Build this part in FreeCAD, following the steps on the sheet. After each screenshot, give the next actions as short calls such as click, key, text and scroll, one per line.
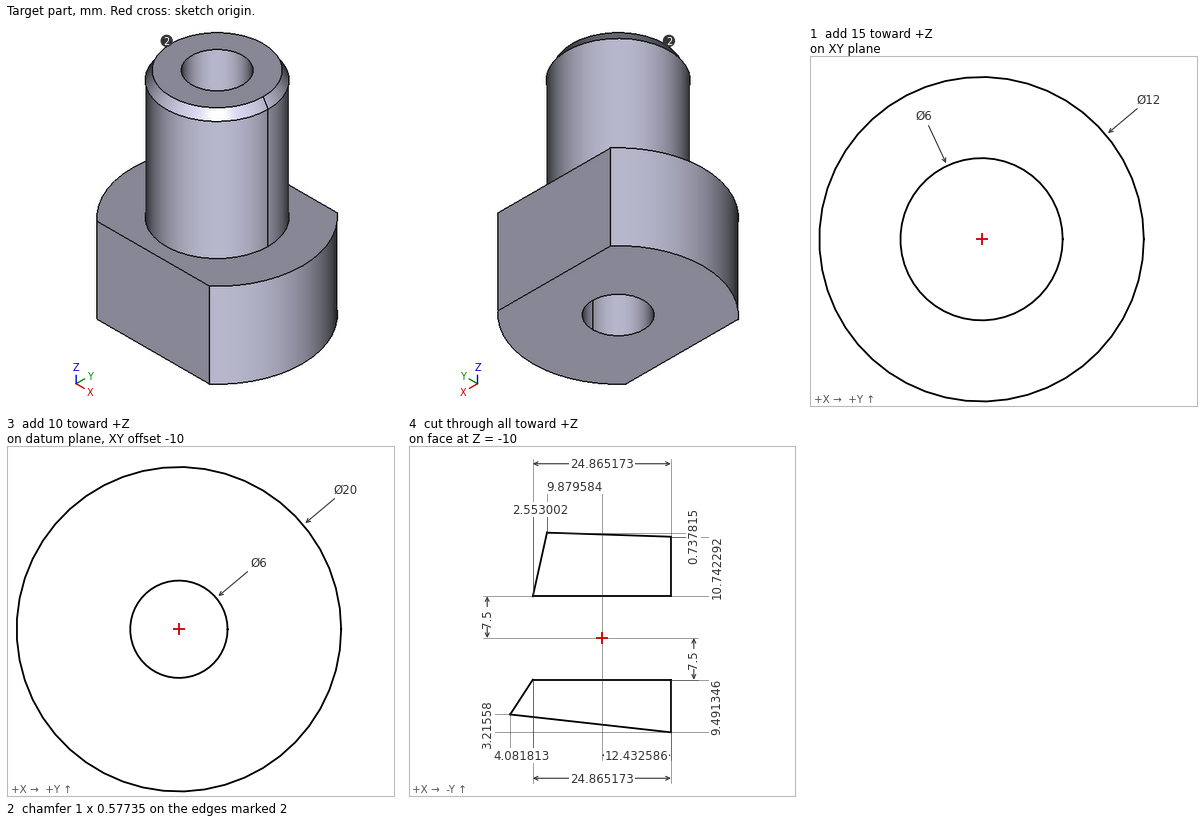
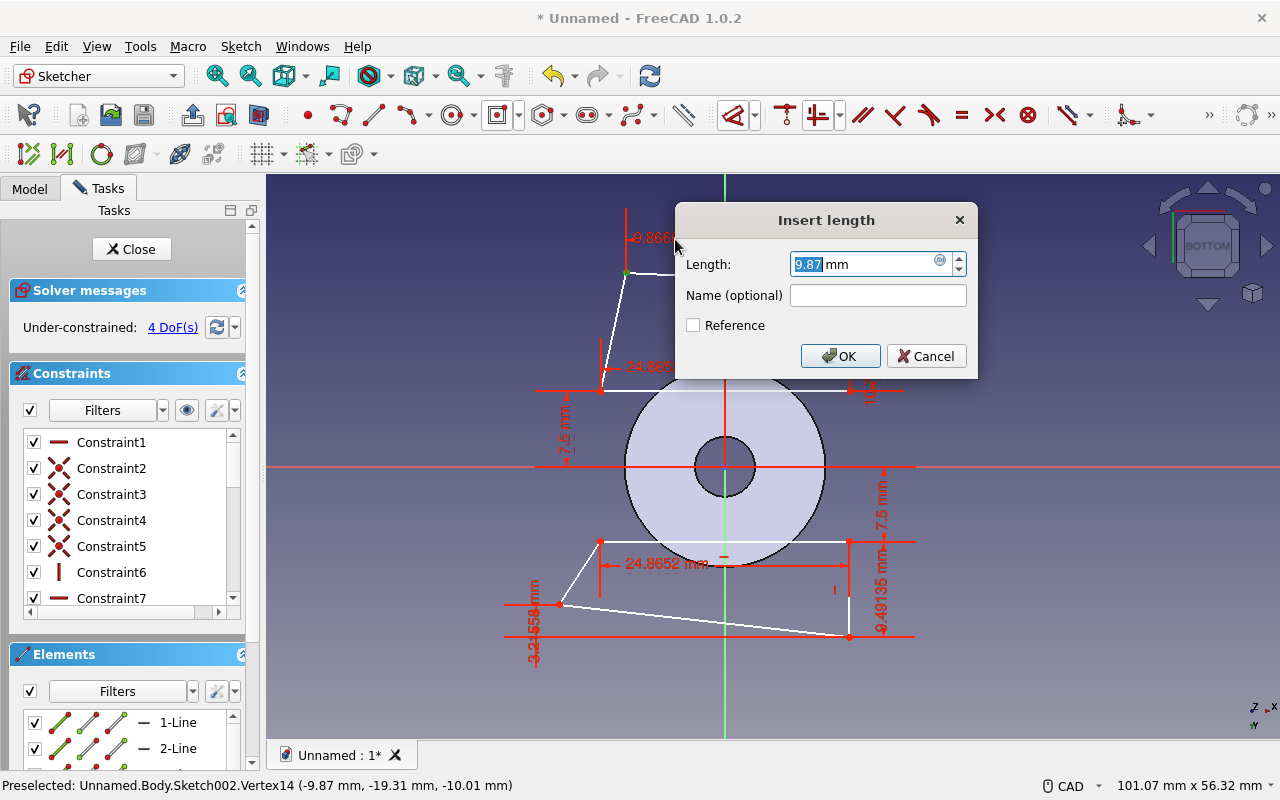
text(9.879584)
key(Return)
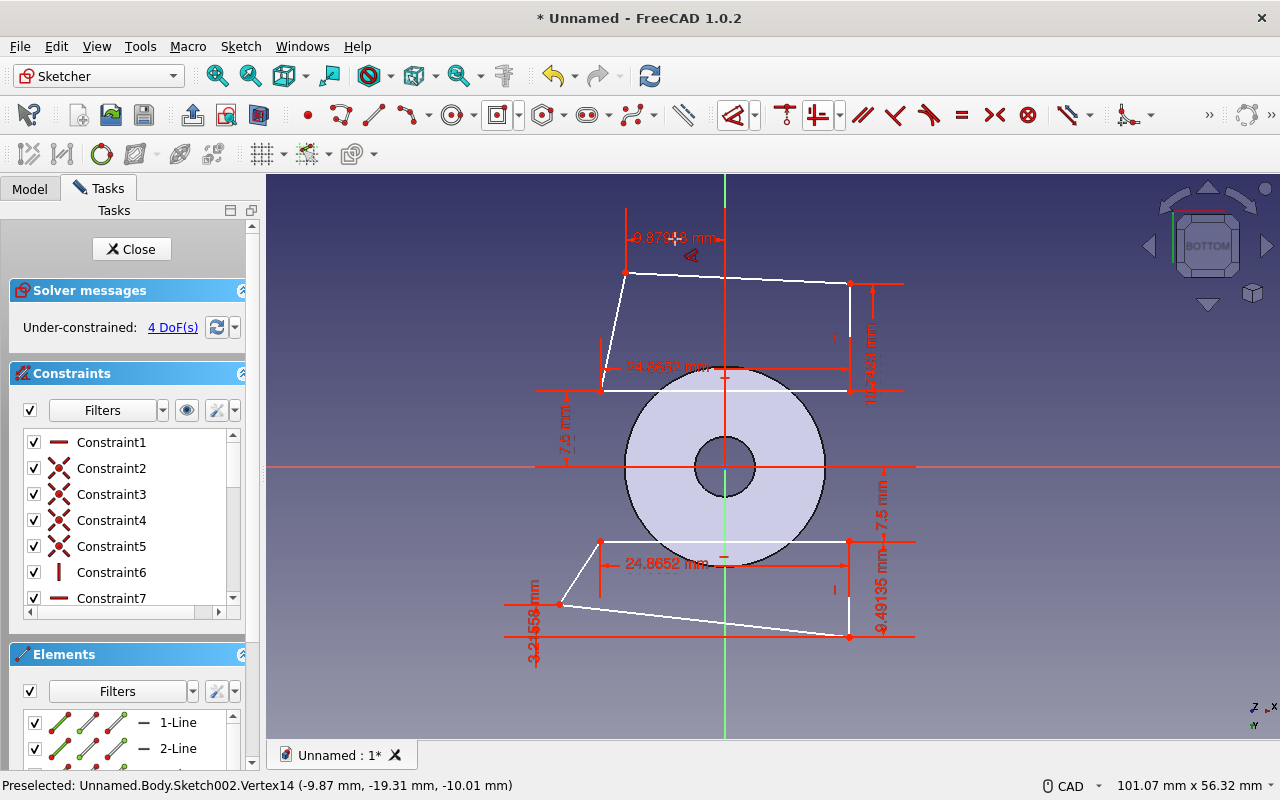
click(588, 561)
click(579, 508)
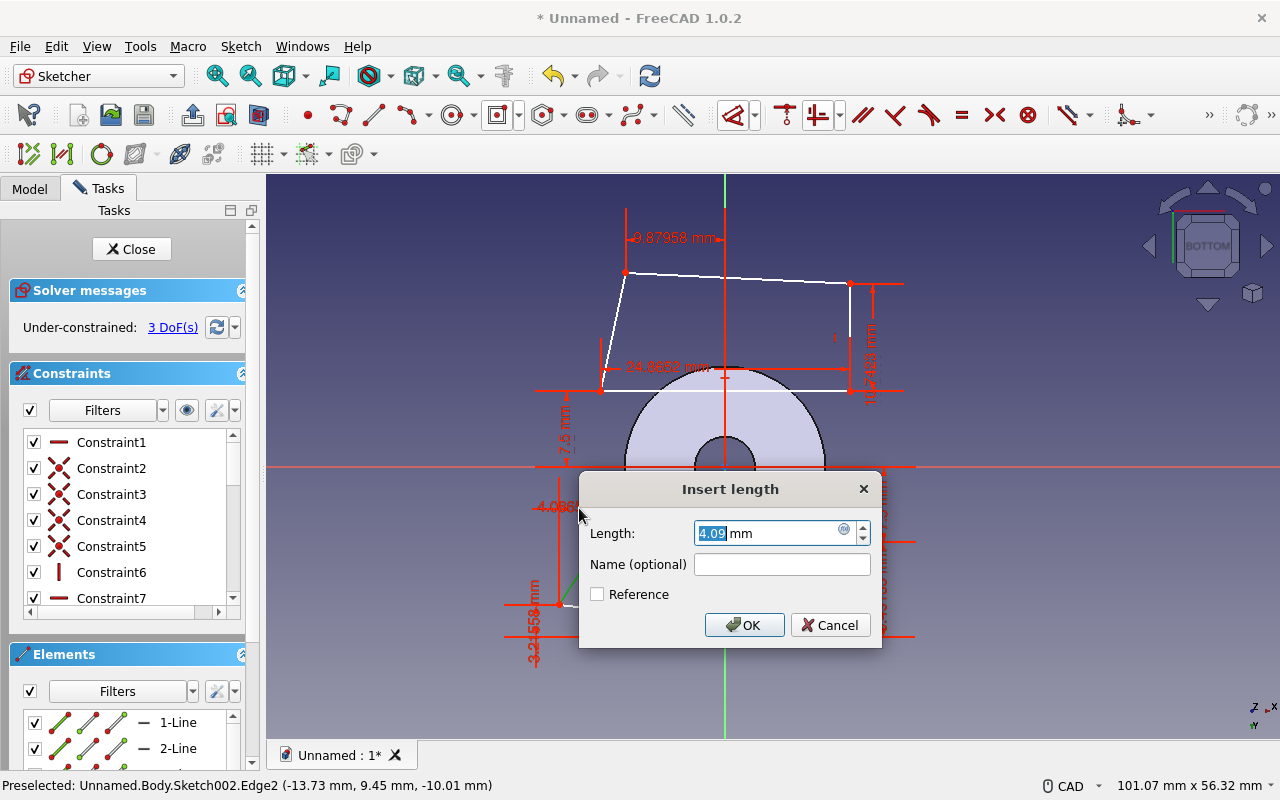
text(4.081813)
key(Return)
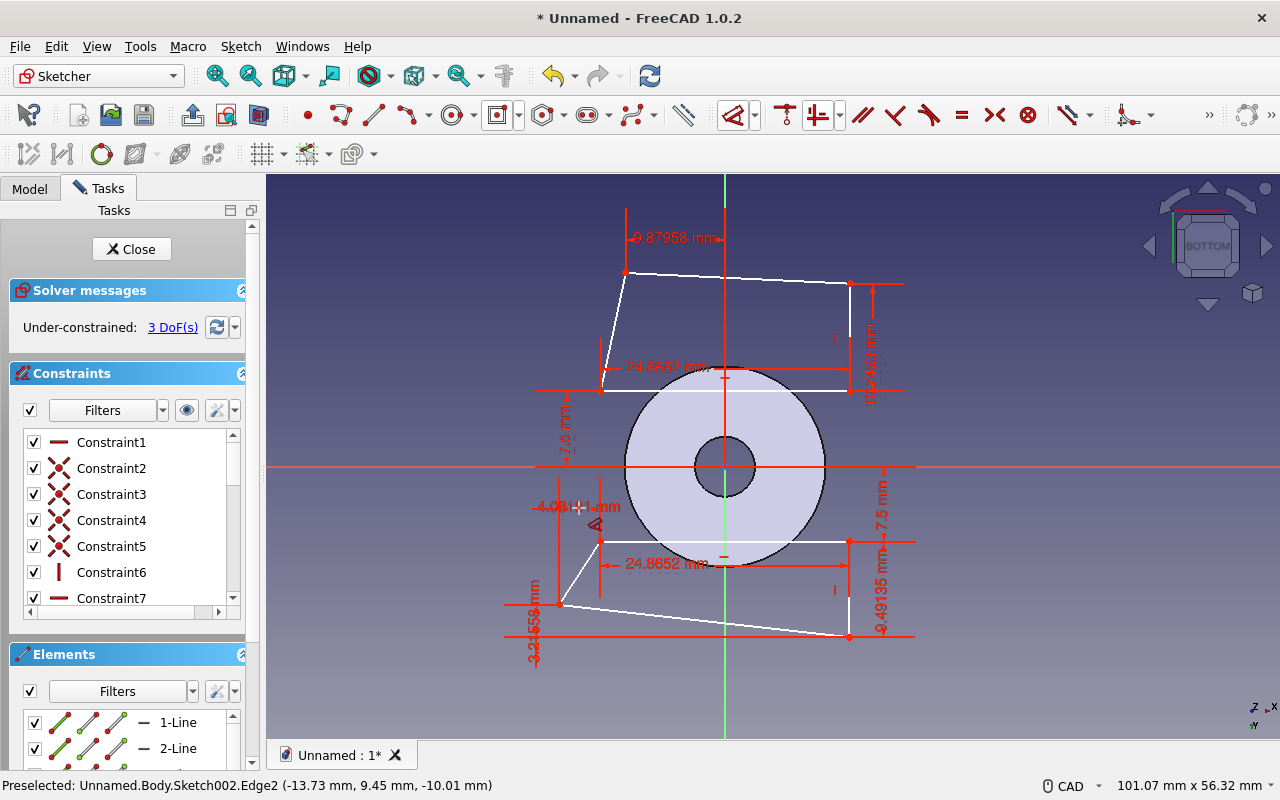
scroll(783, 281, up, 9)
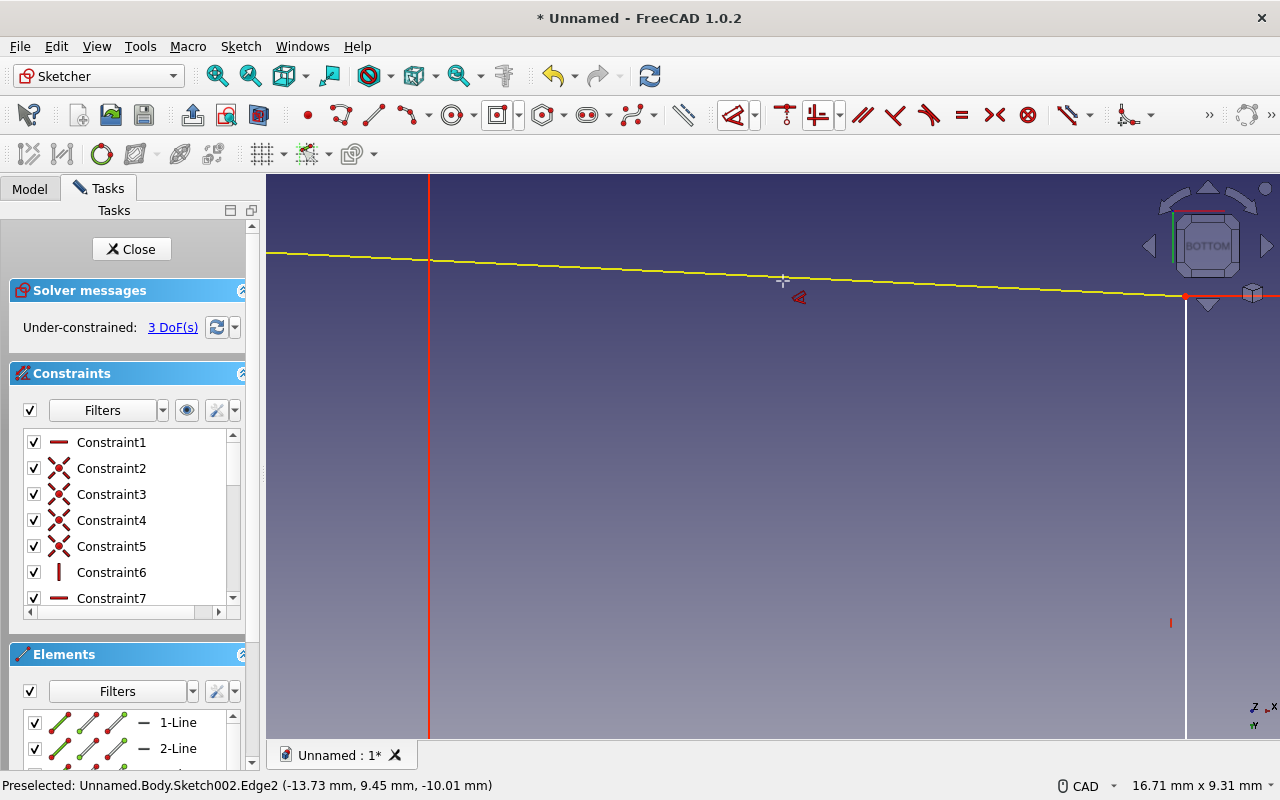
click(779, 277)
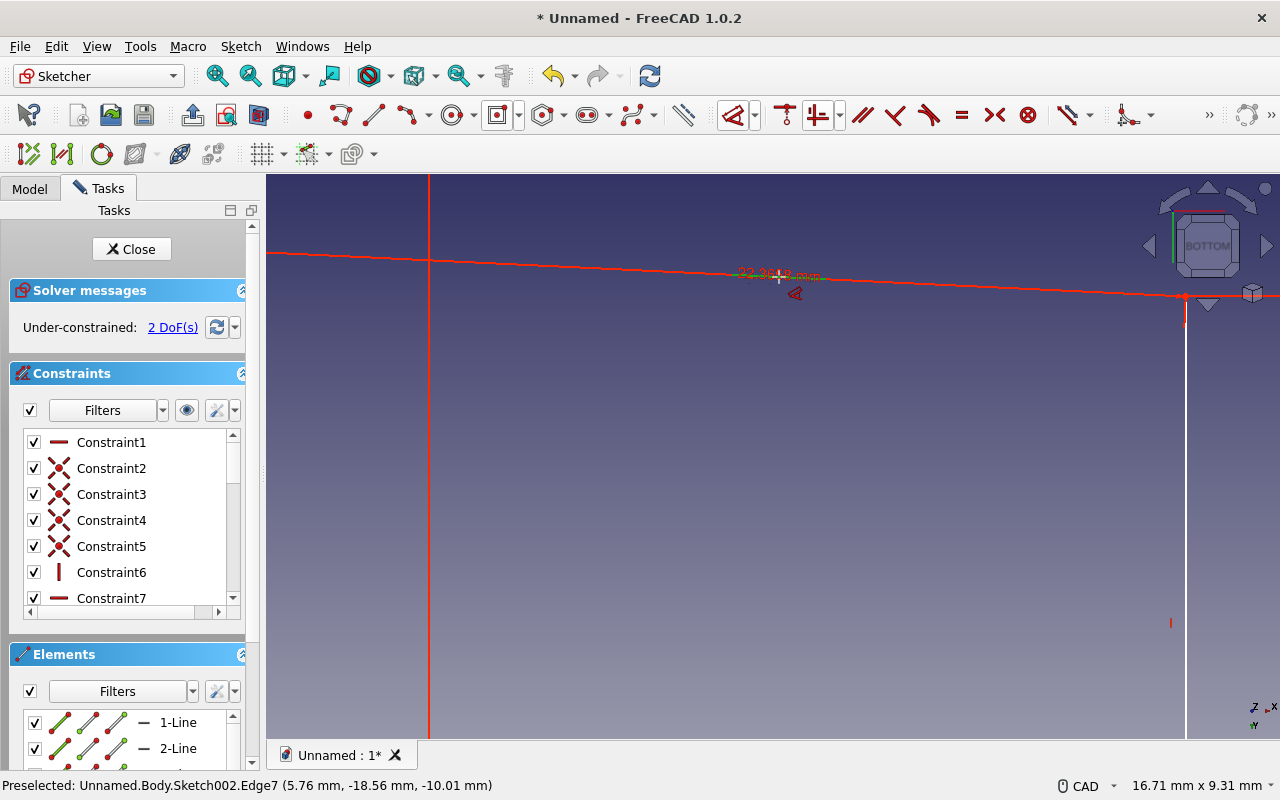
key(Escape)
key(Escape)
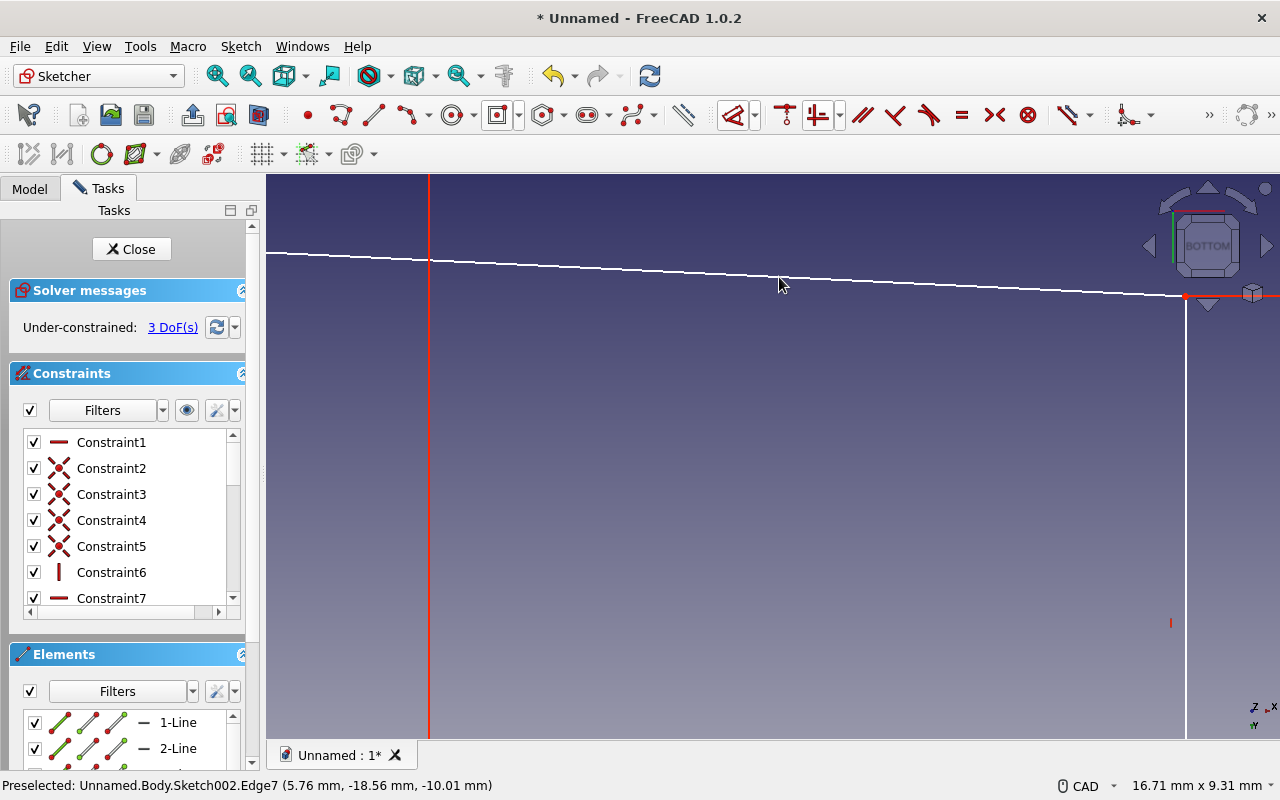
click(779, 277)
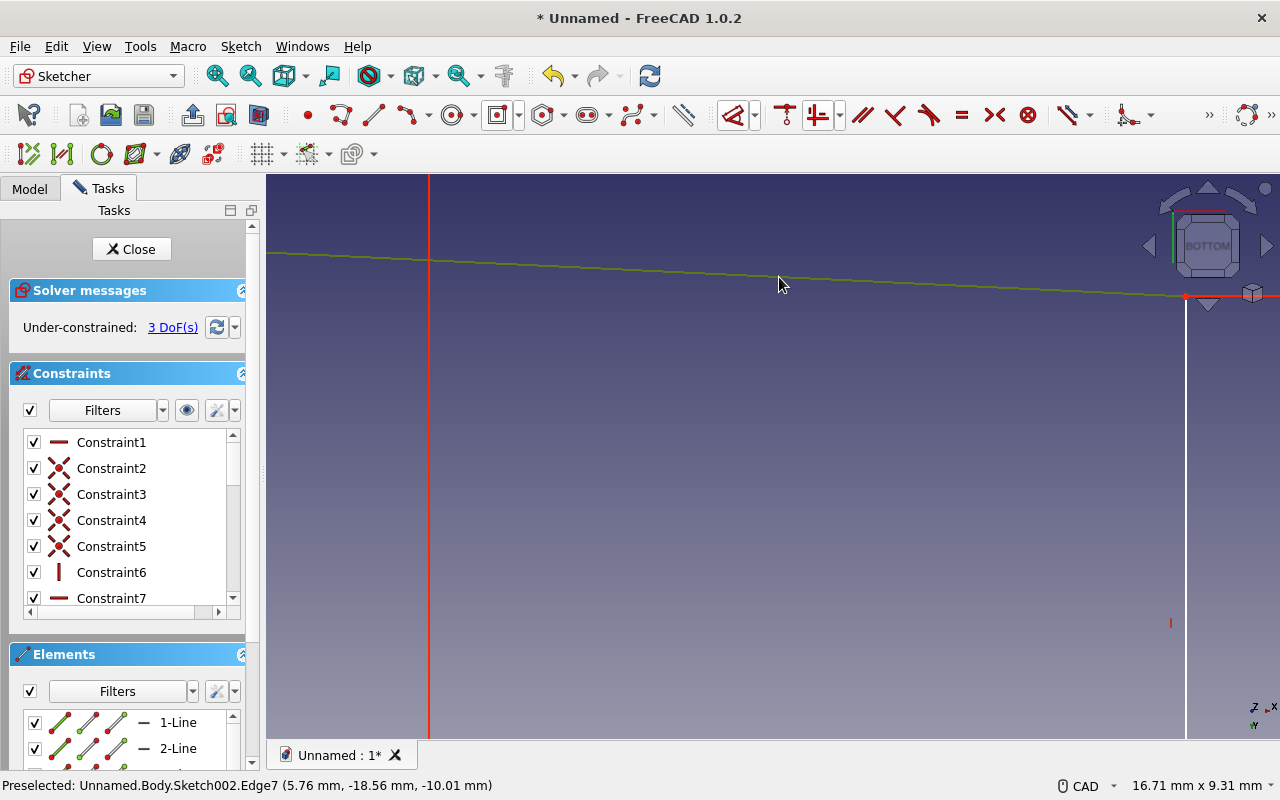
click(754, 116)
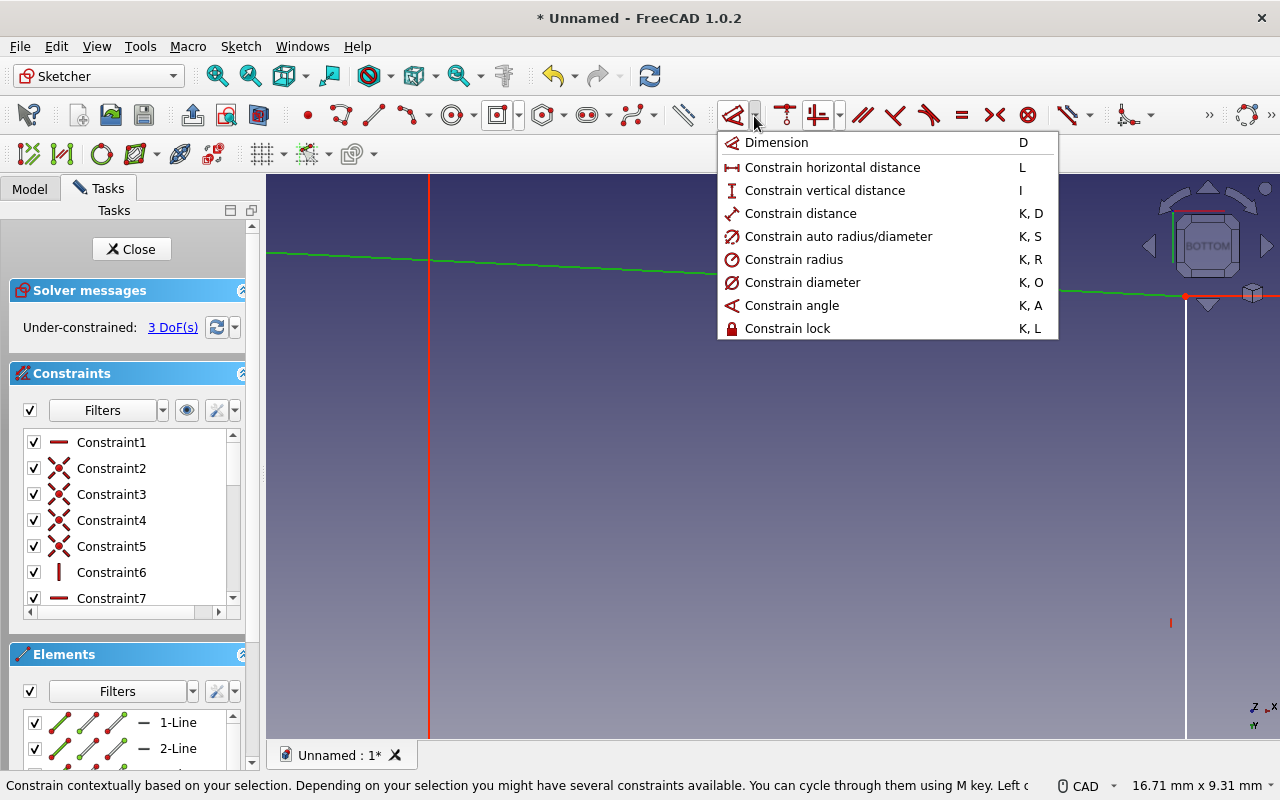
click(888, 190)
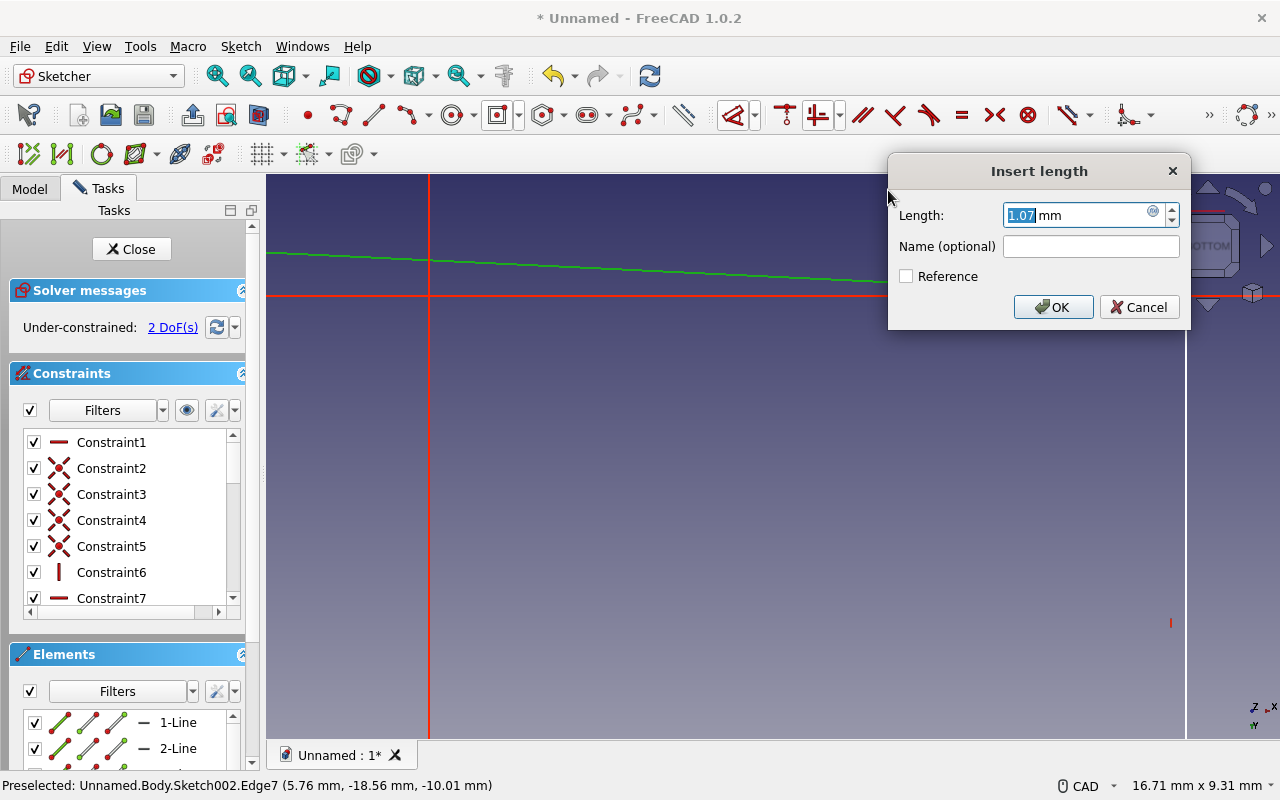
text(0.737815)
key(Return)